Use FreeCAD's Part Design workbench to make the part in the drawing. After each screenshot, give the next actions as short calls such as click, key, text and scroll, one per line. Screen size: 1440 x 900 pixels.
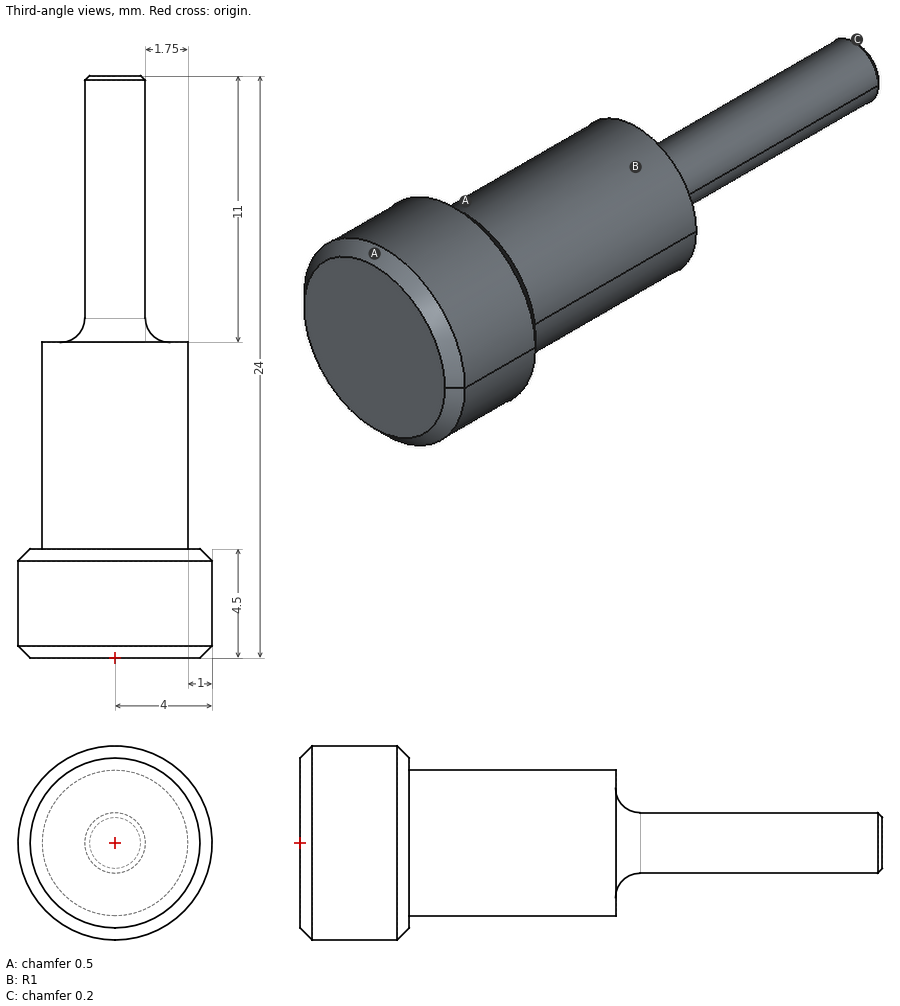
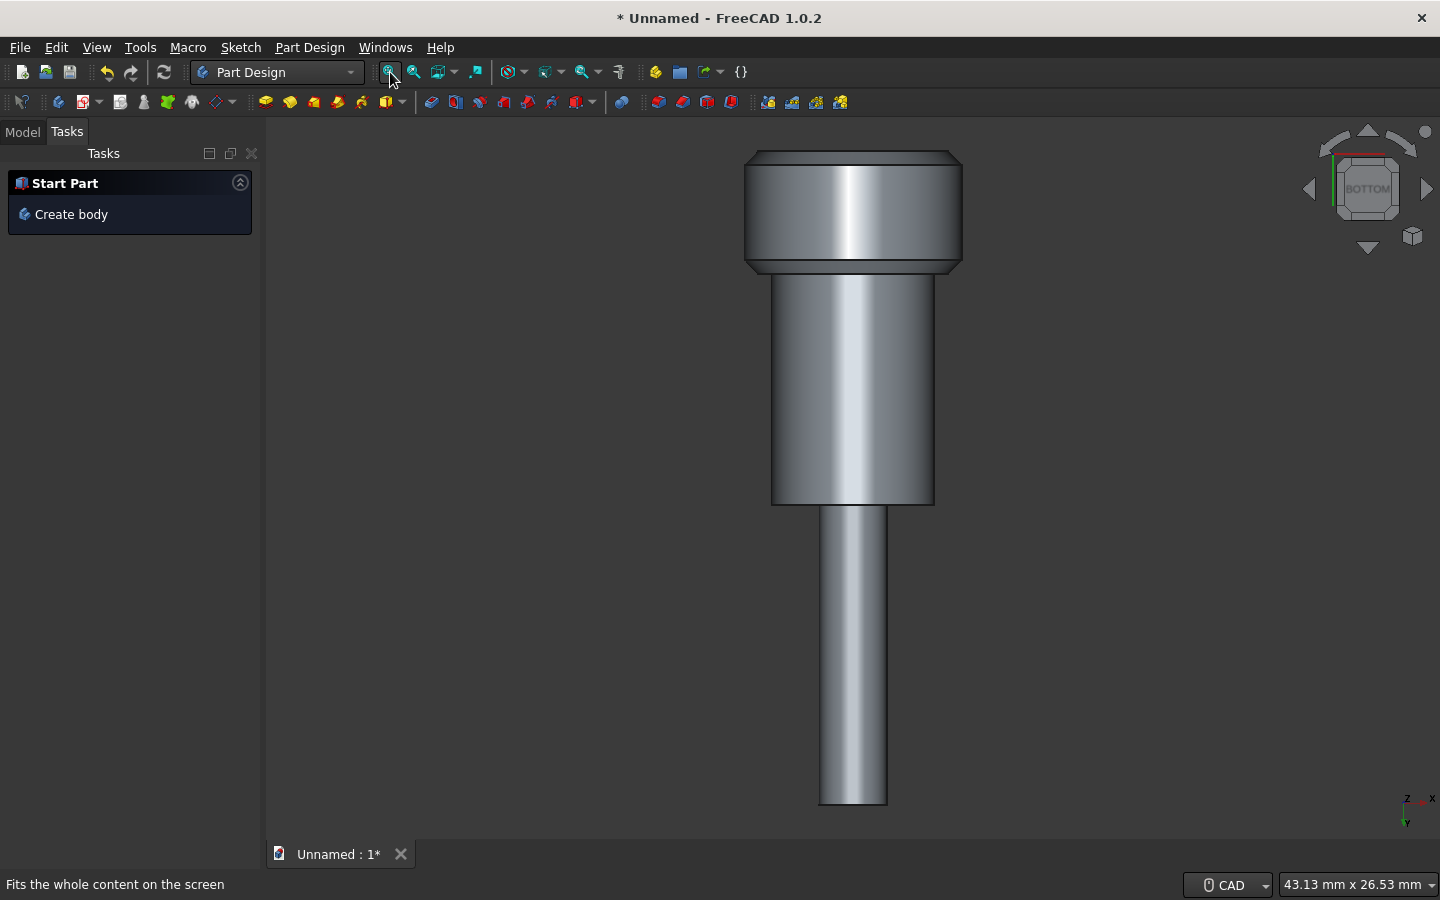
key(4)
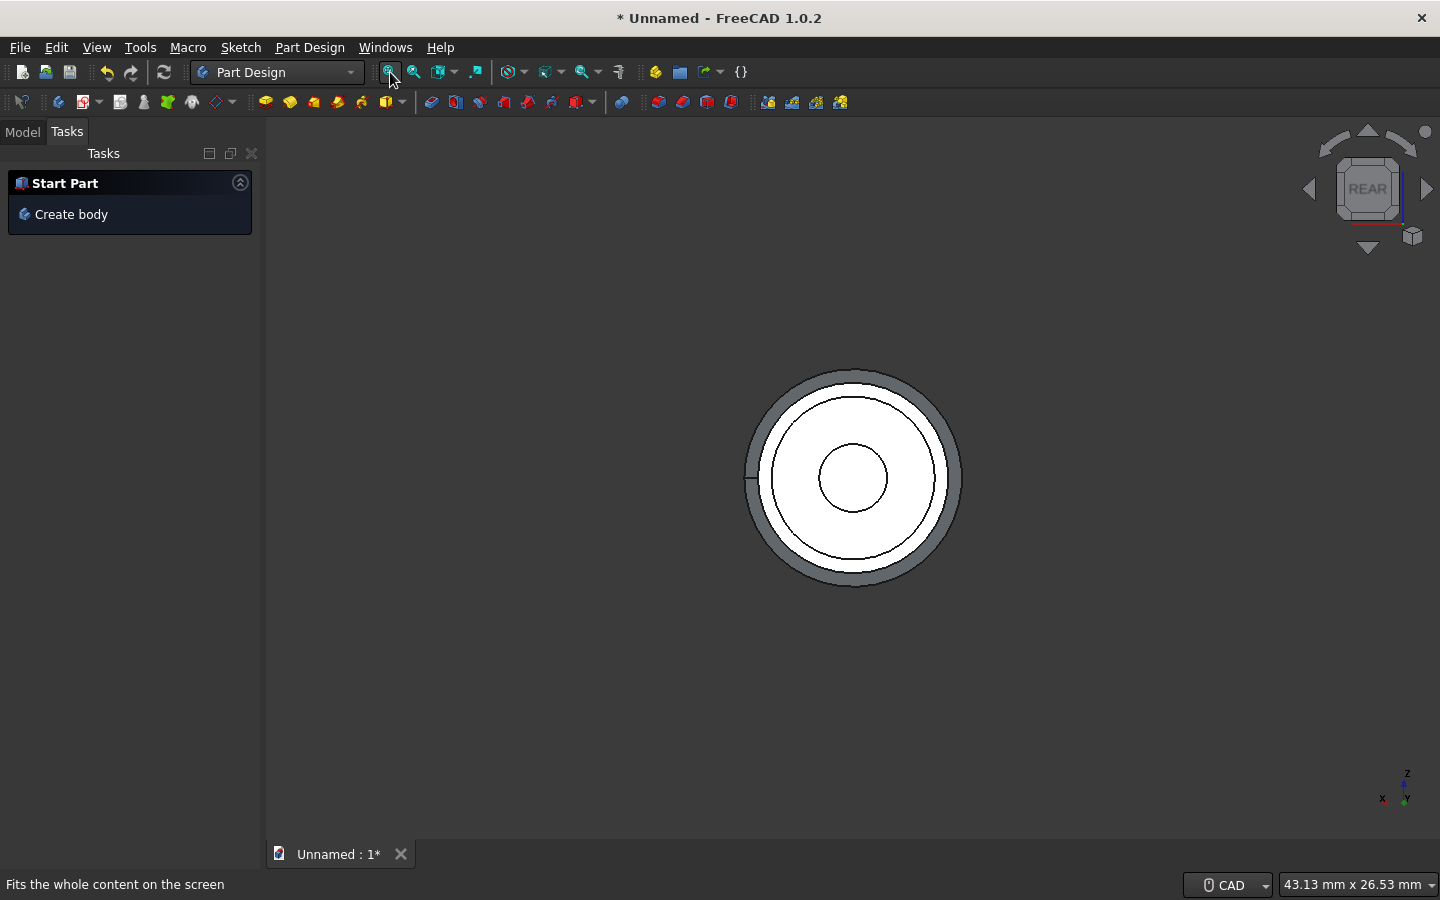
click(390, 72)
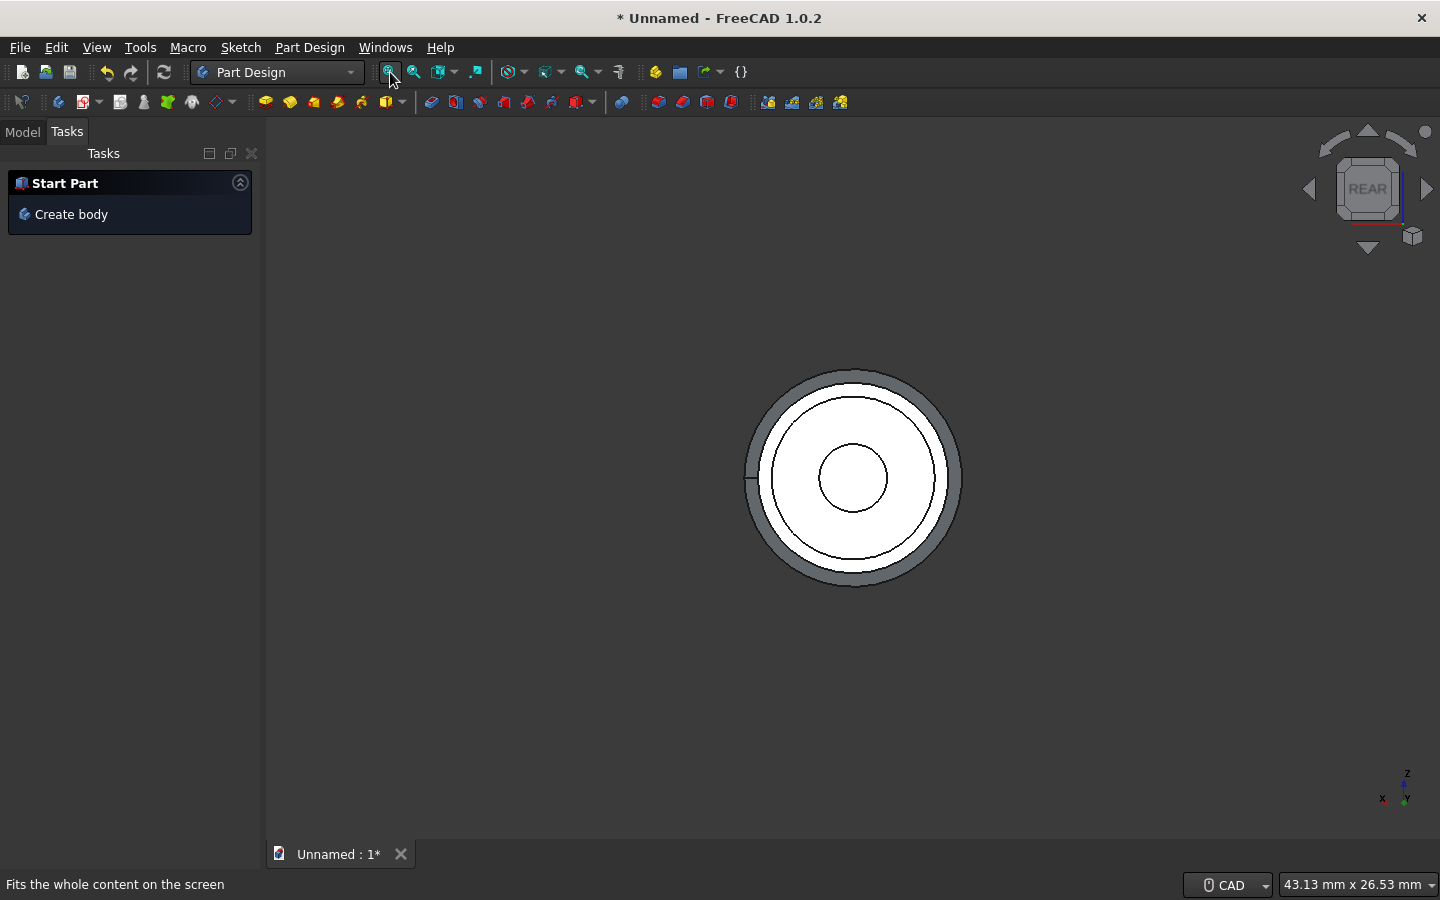
key(6)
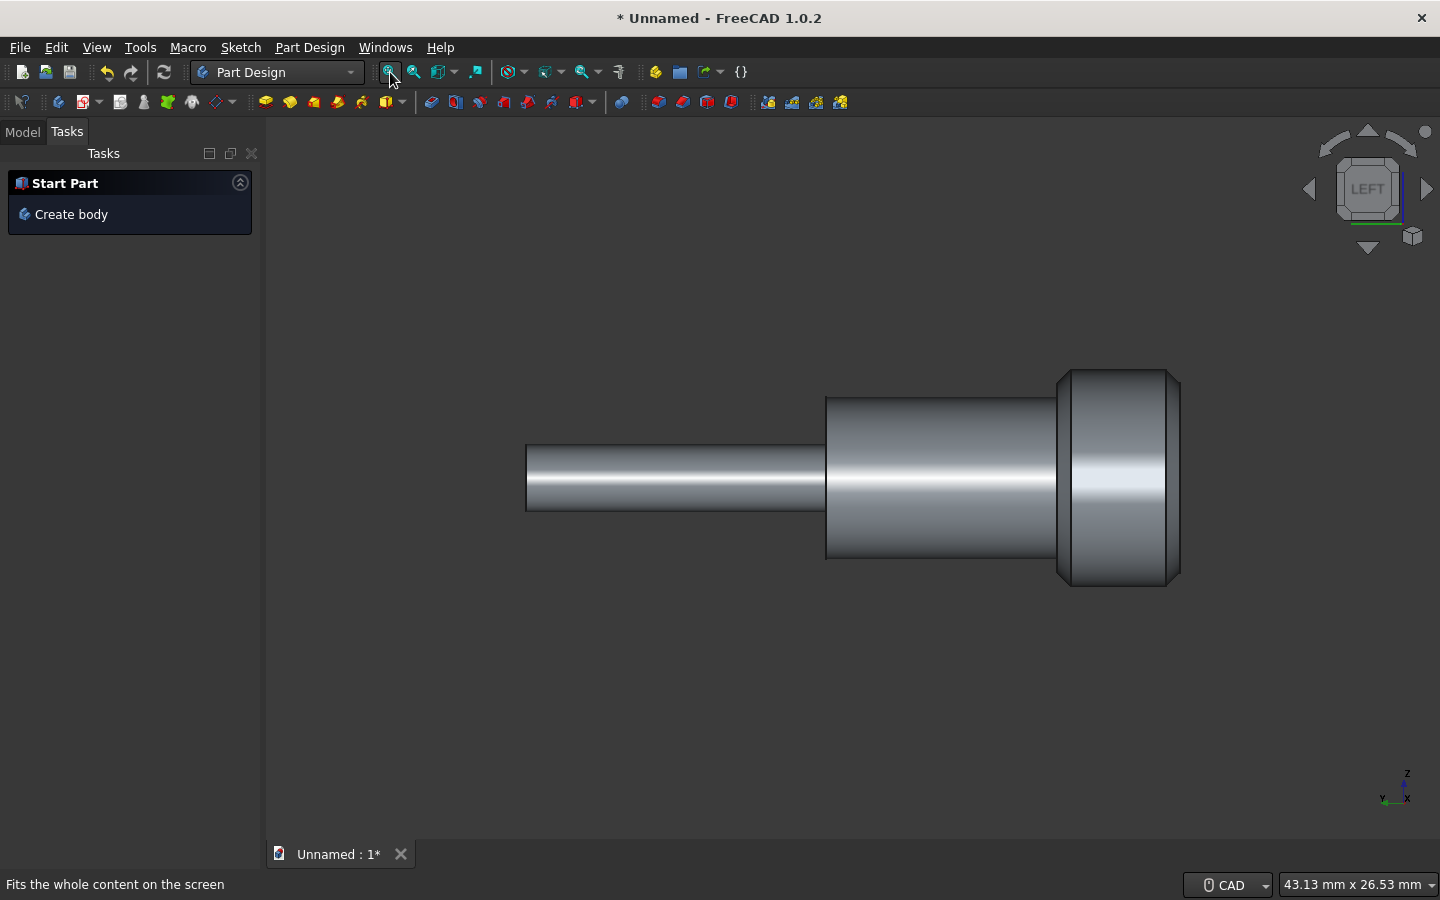
key(v)
key(3)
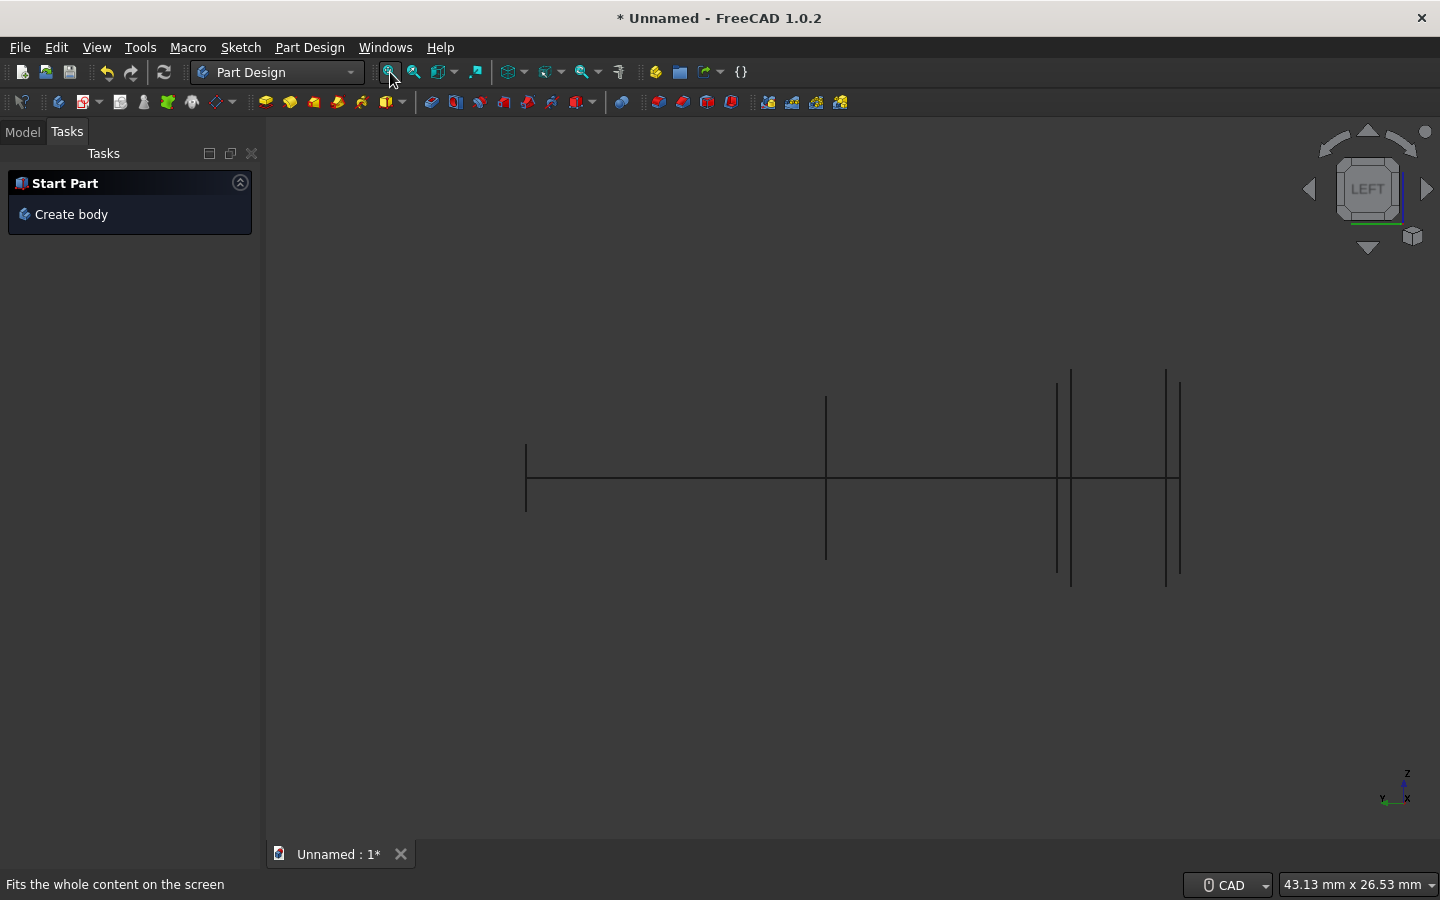
key(0)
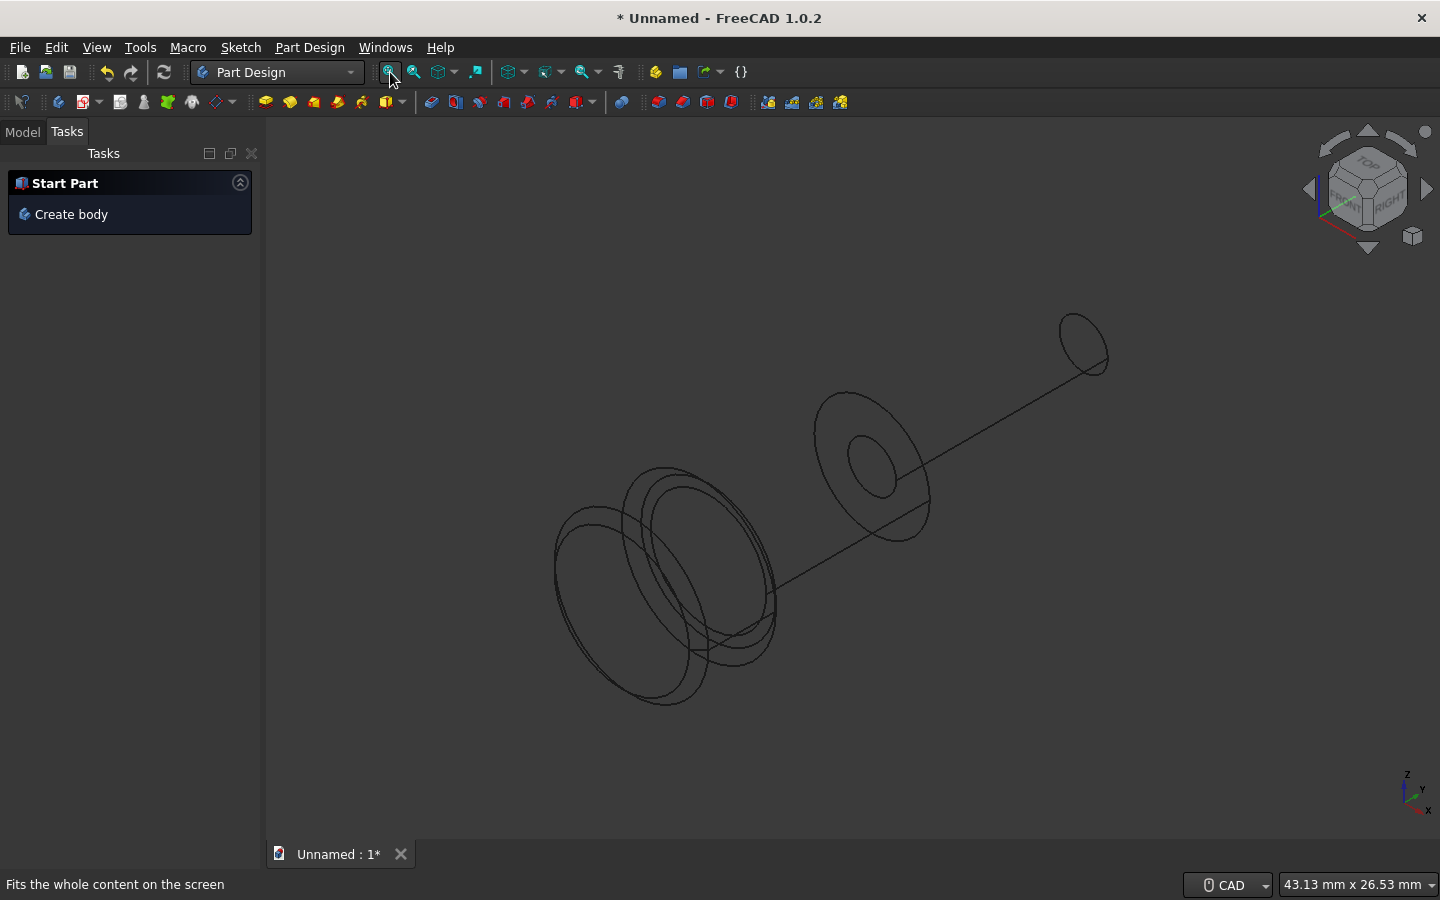
click(848, 452)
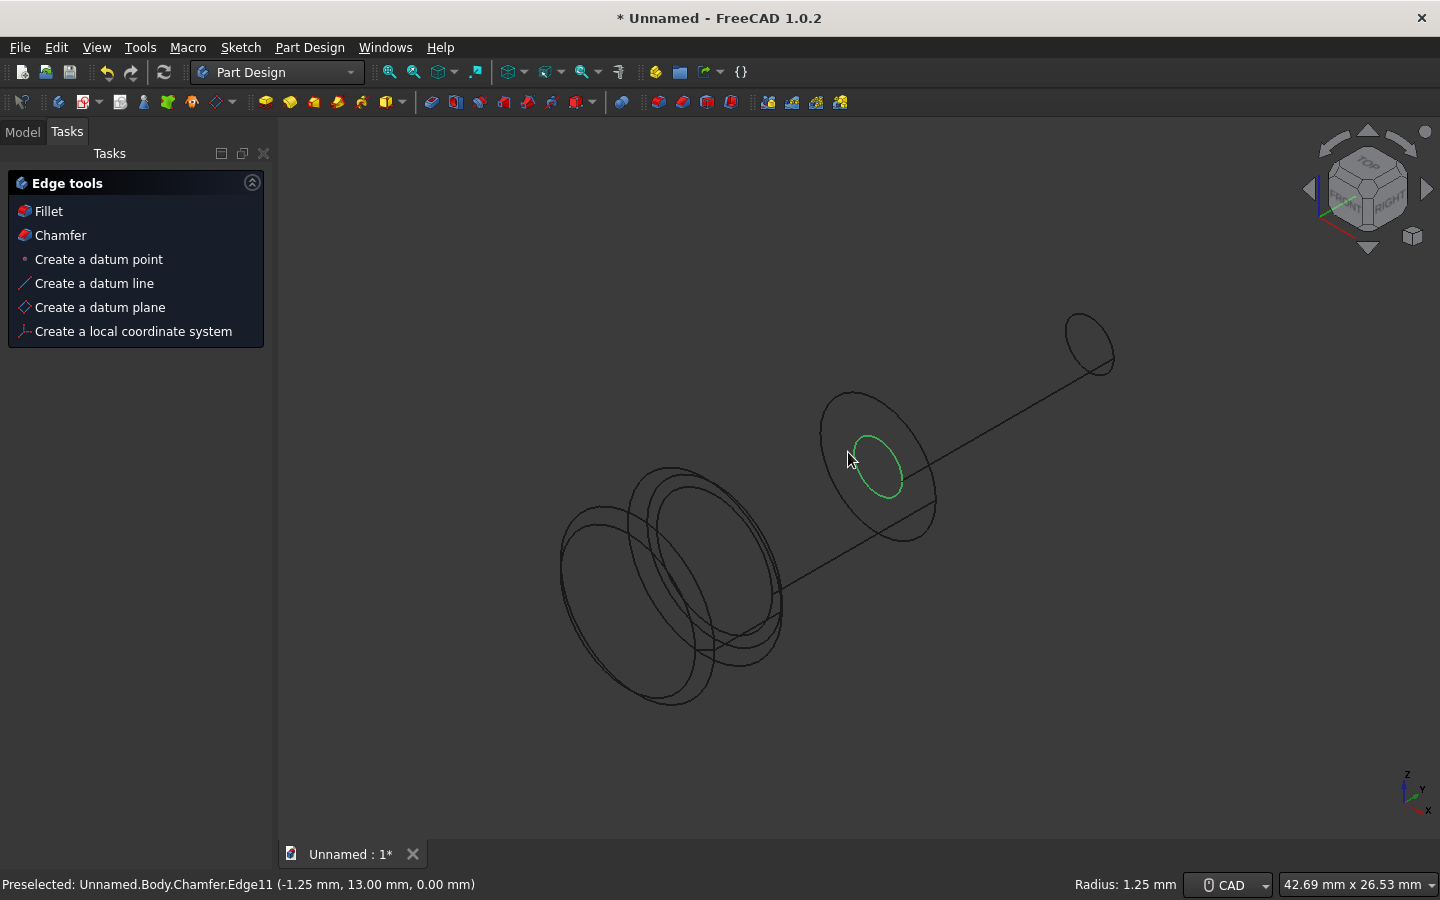
key(v)
key(1)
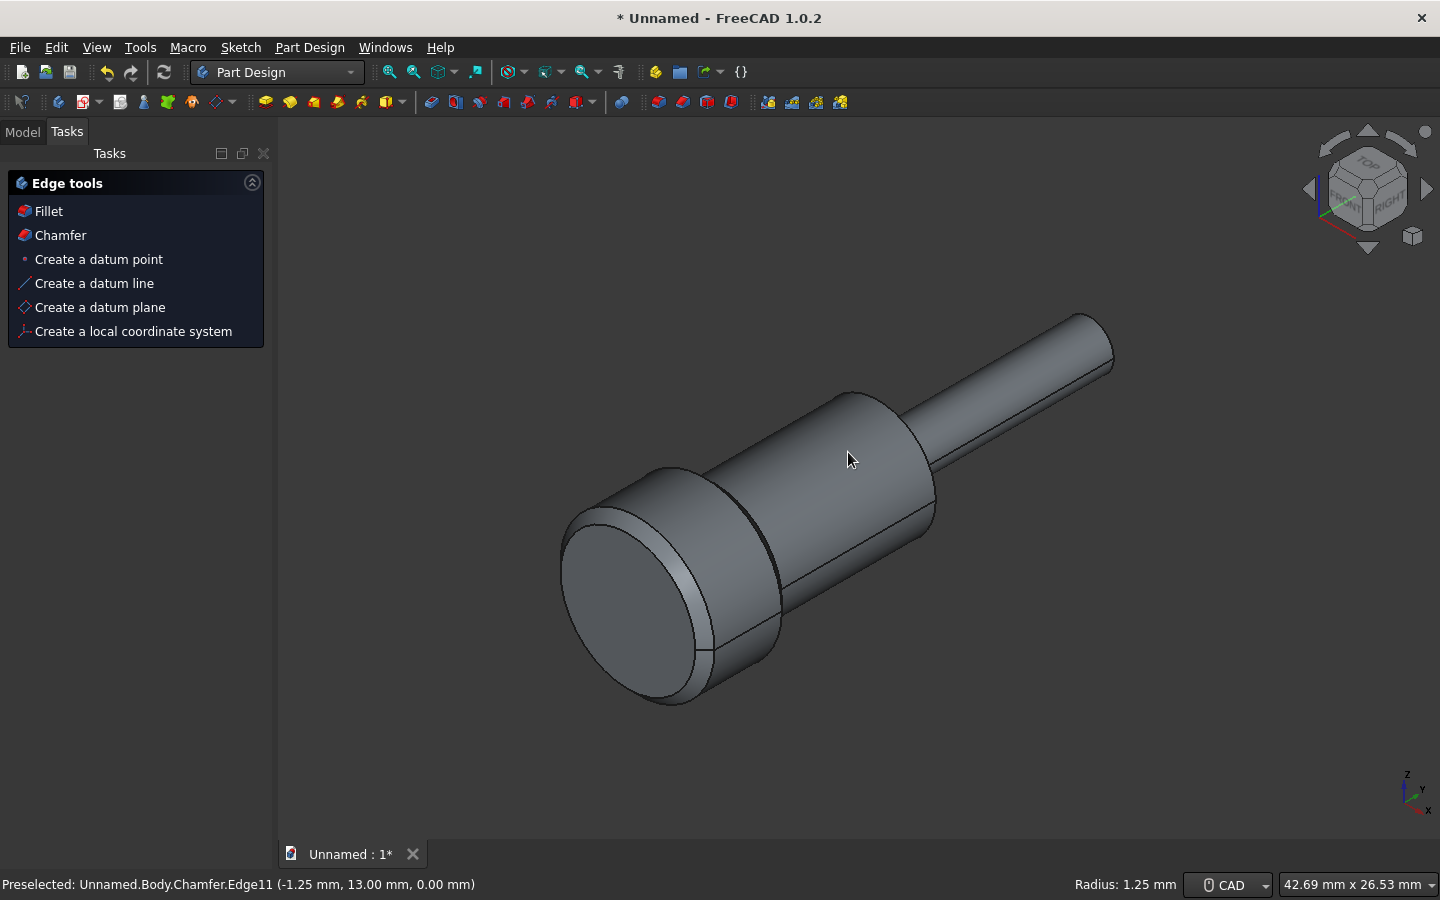
click(660, 102)